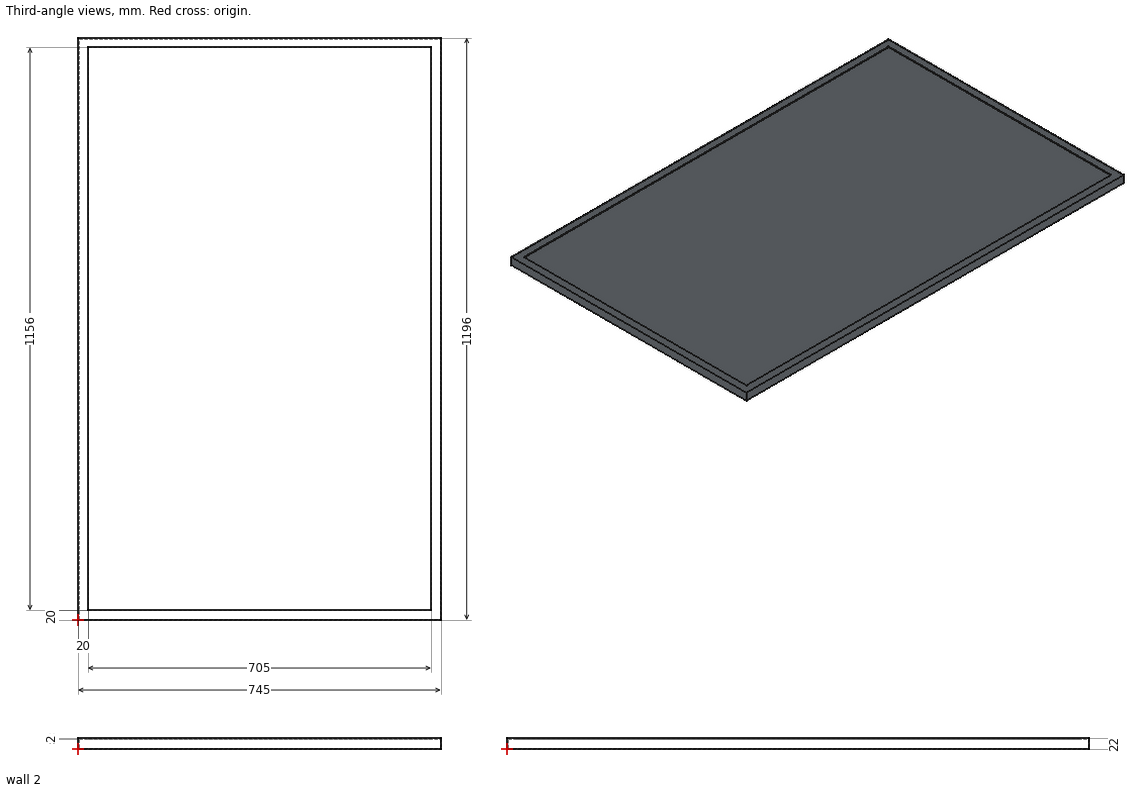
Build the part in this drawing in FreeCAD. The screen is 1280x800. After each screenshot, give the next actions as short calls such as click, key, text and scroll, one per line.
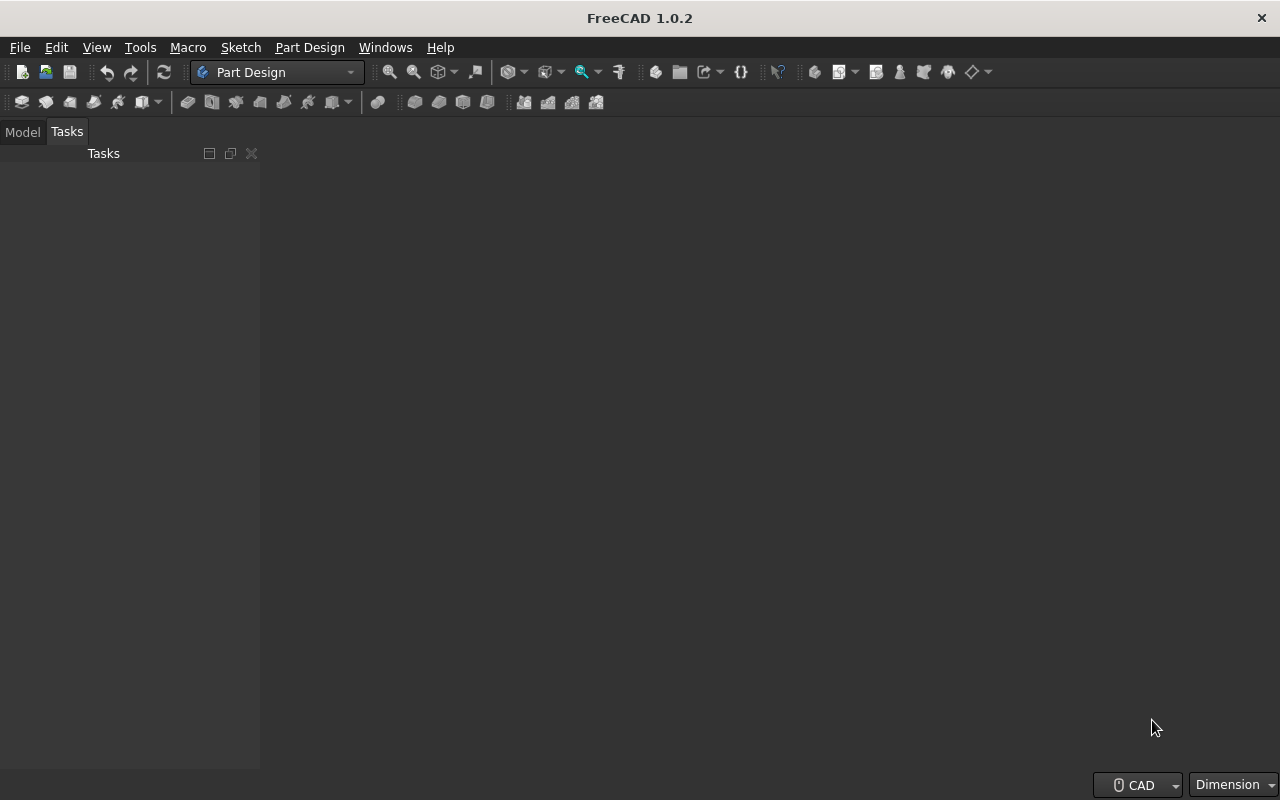
click(22, 72)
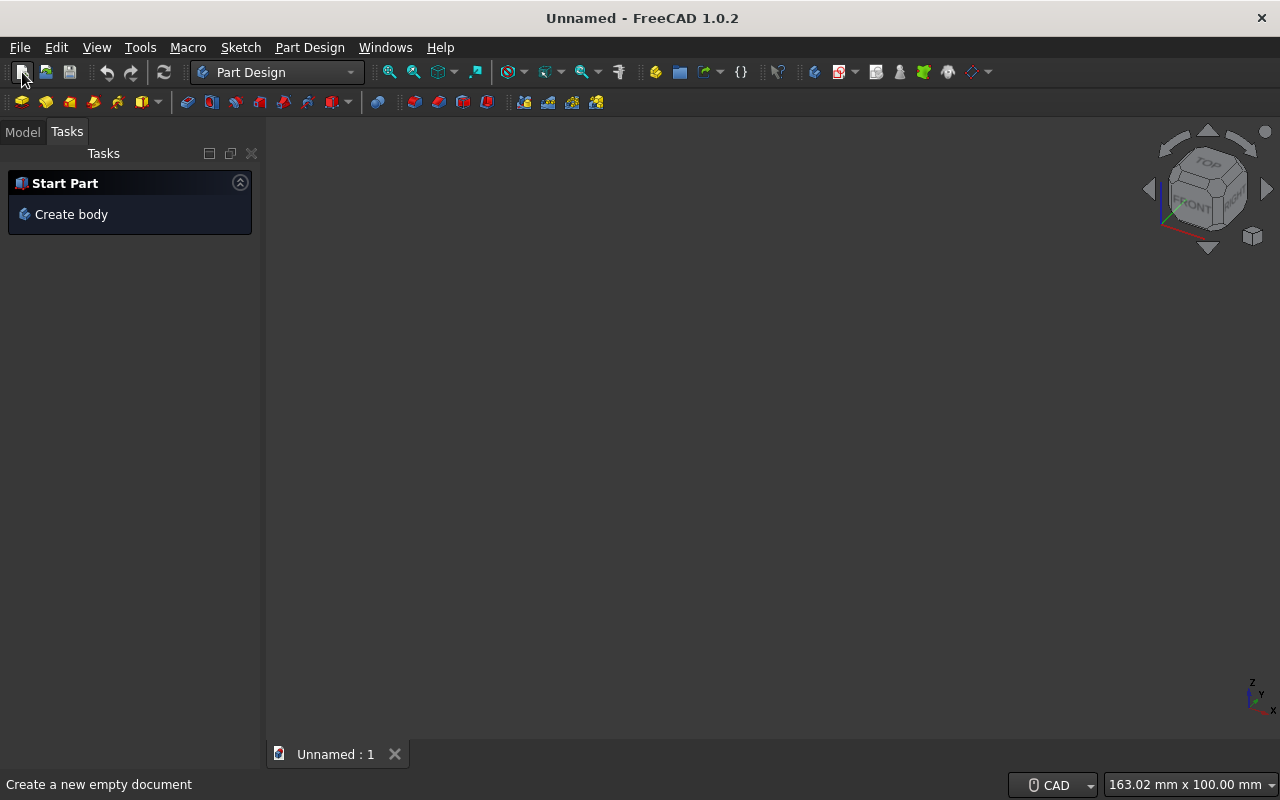
click(840, 72)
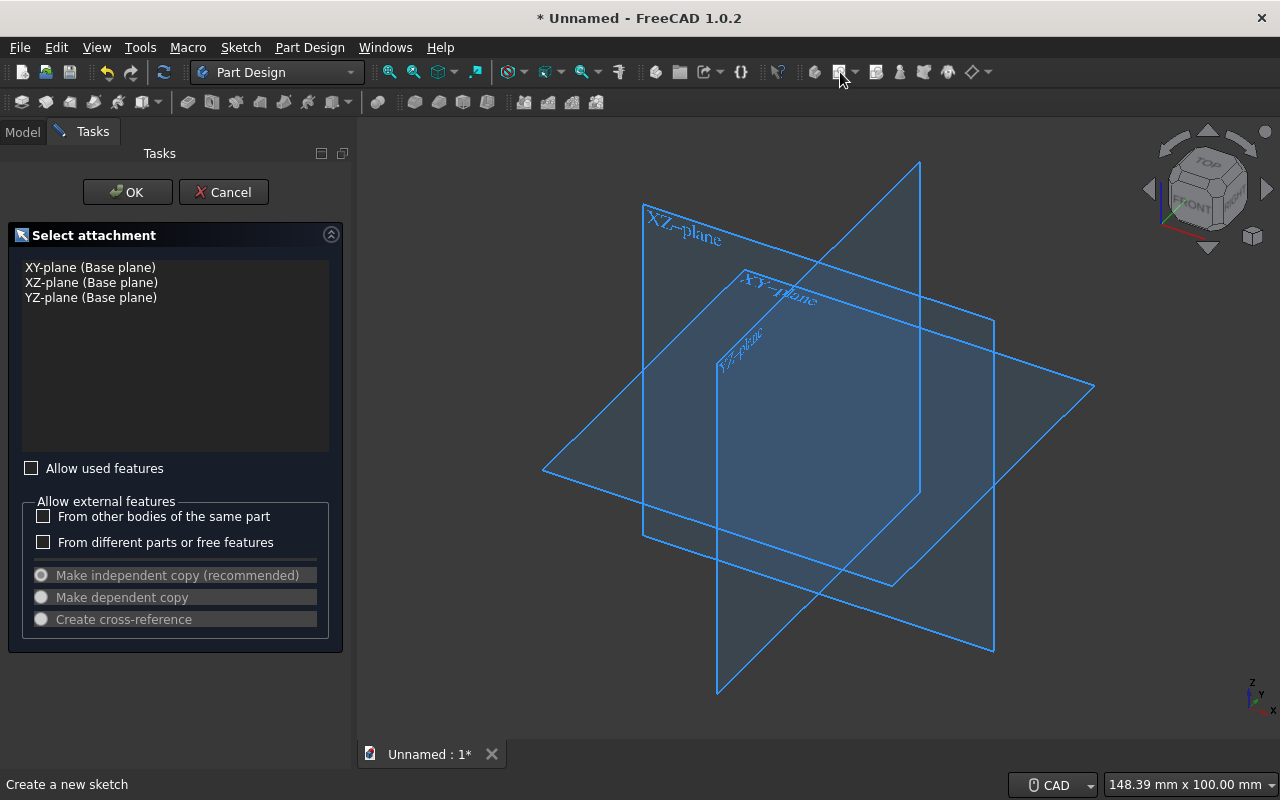
click(82, 268)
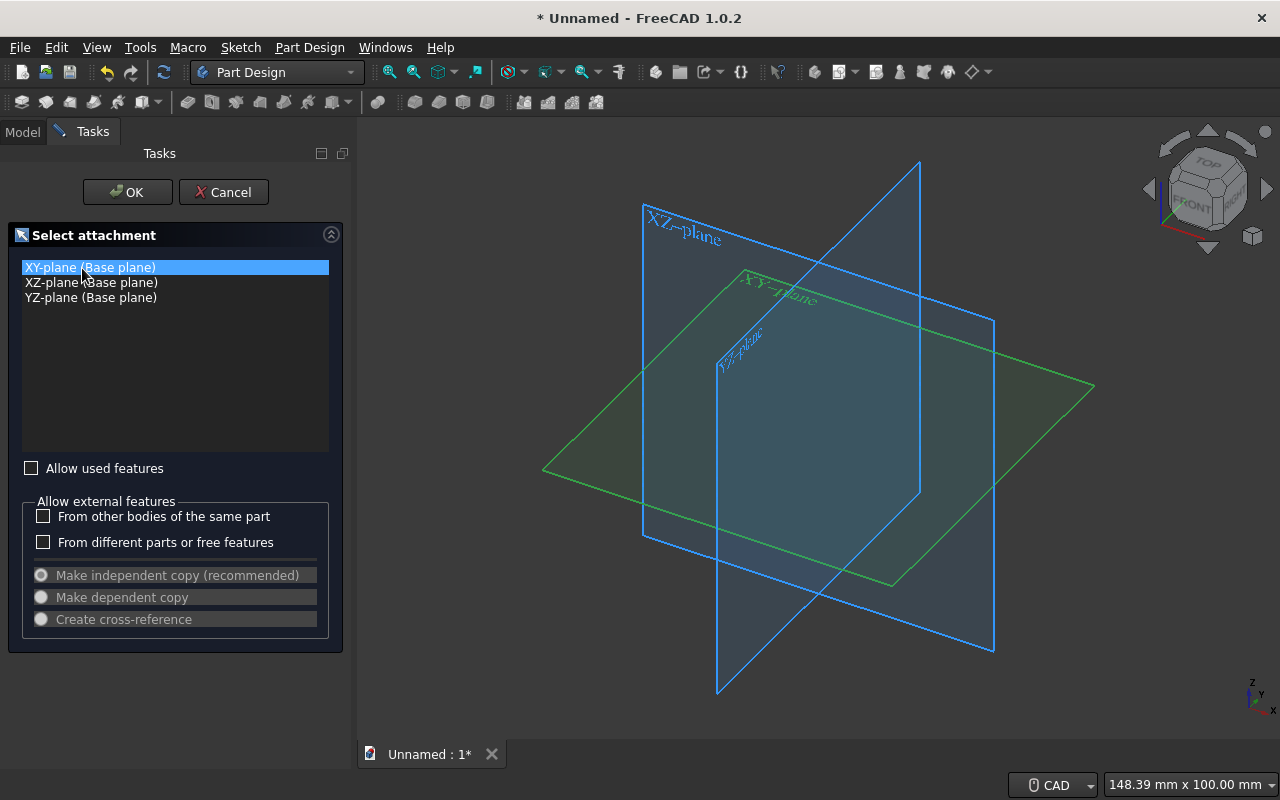
click(128, 192)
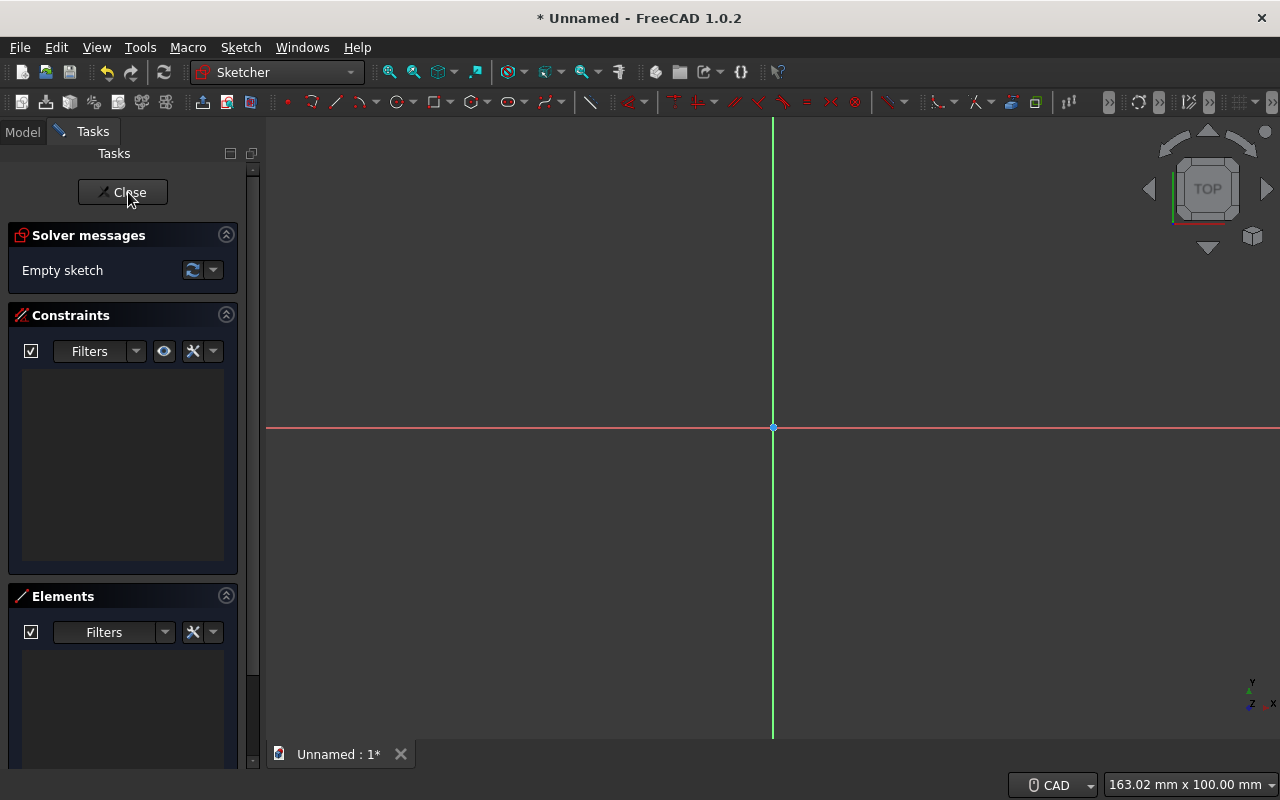
scroll(580, 623, down, 15)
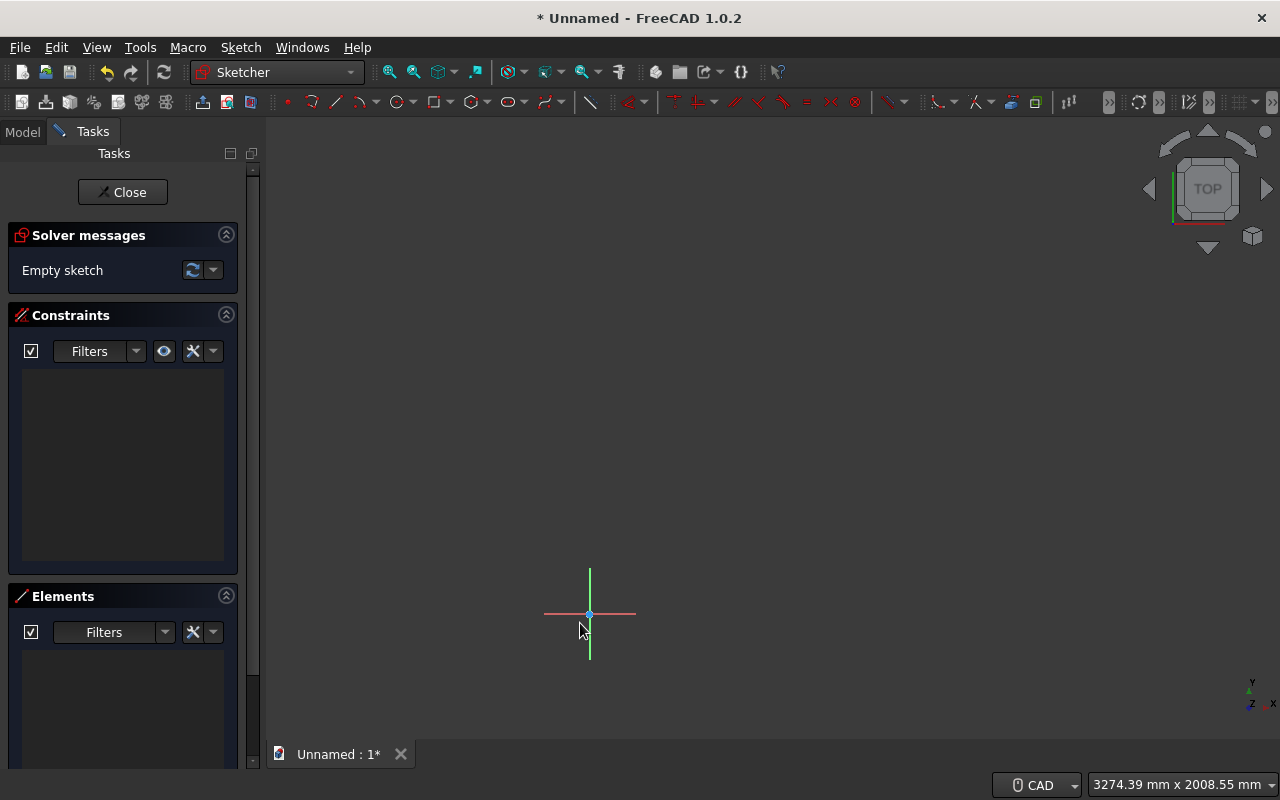
click(434, 102)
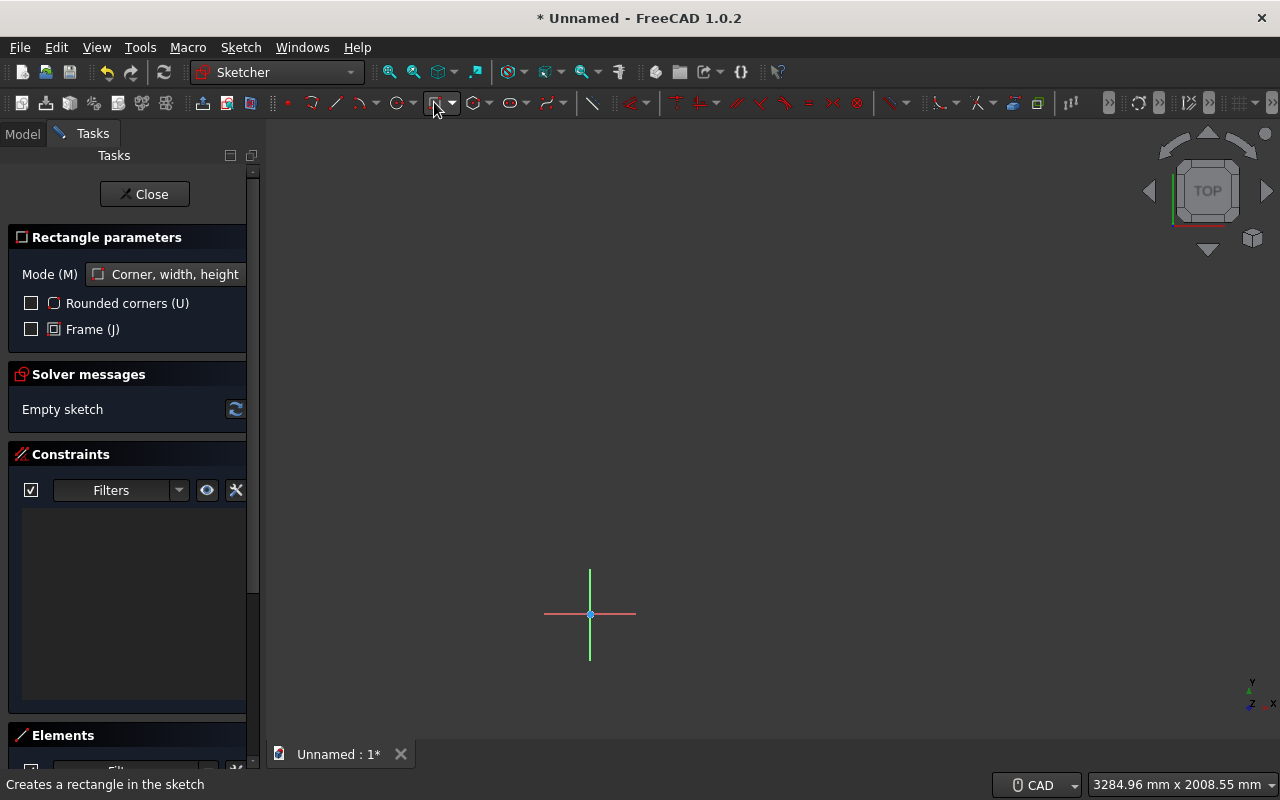
click(590, 614)
move(820, 245)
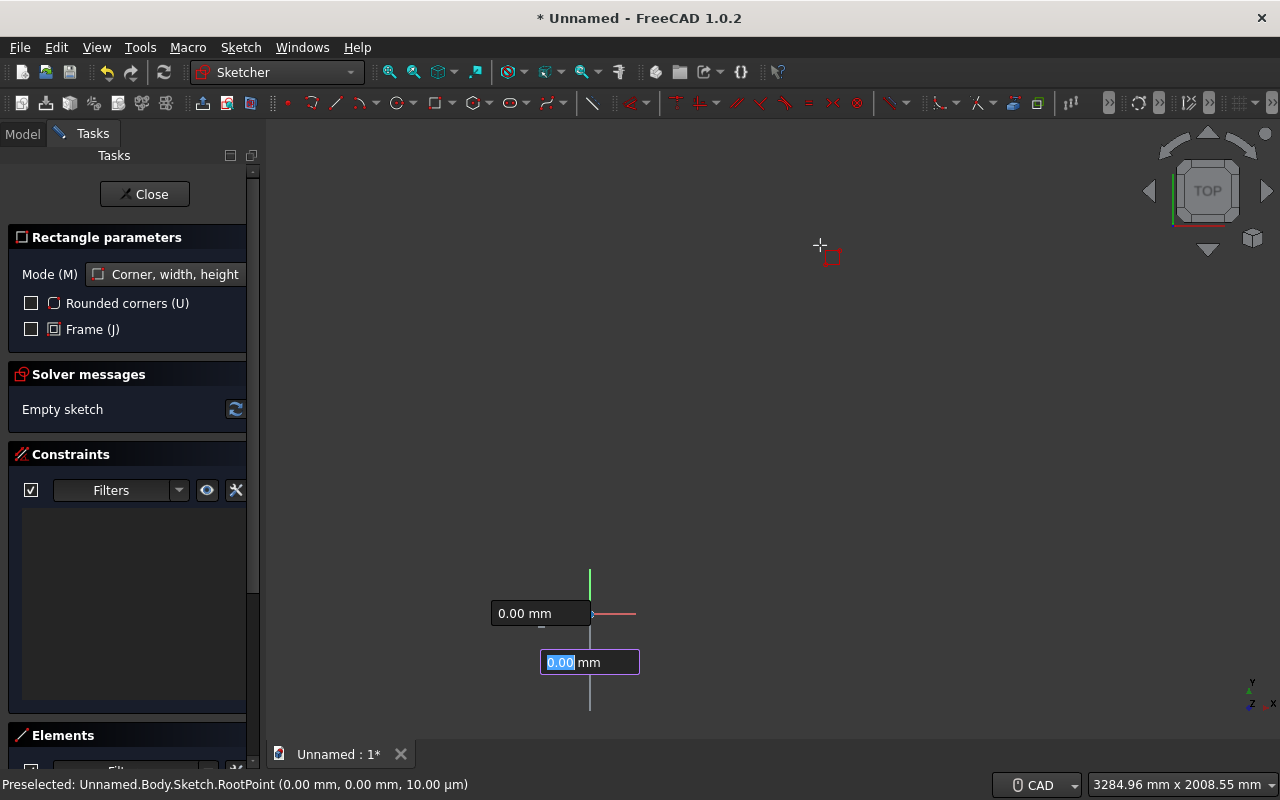
text(745)
key(Tab)
text(1196)
key(Return)
key(Escape)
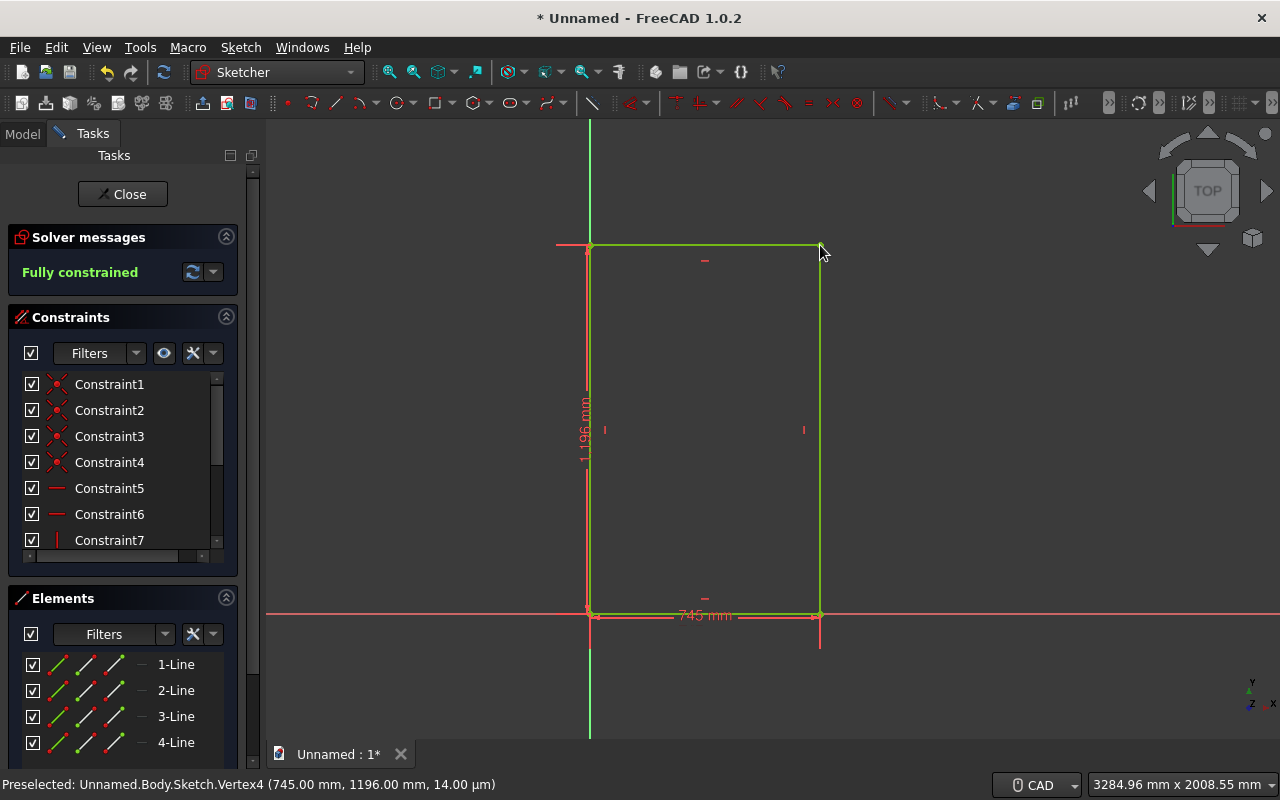
click(123, 194)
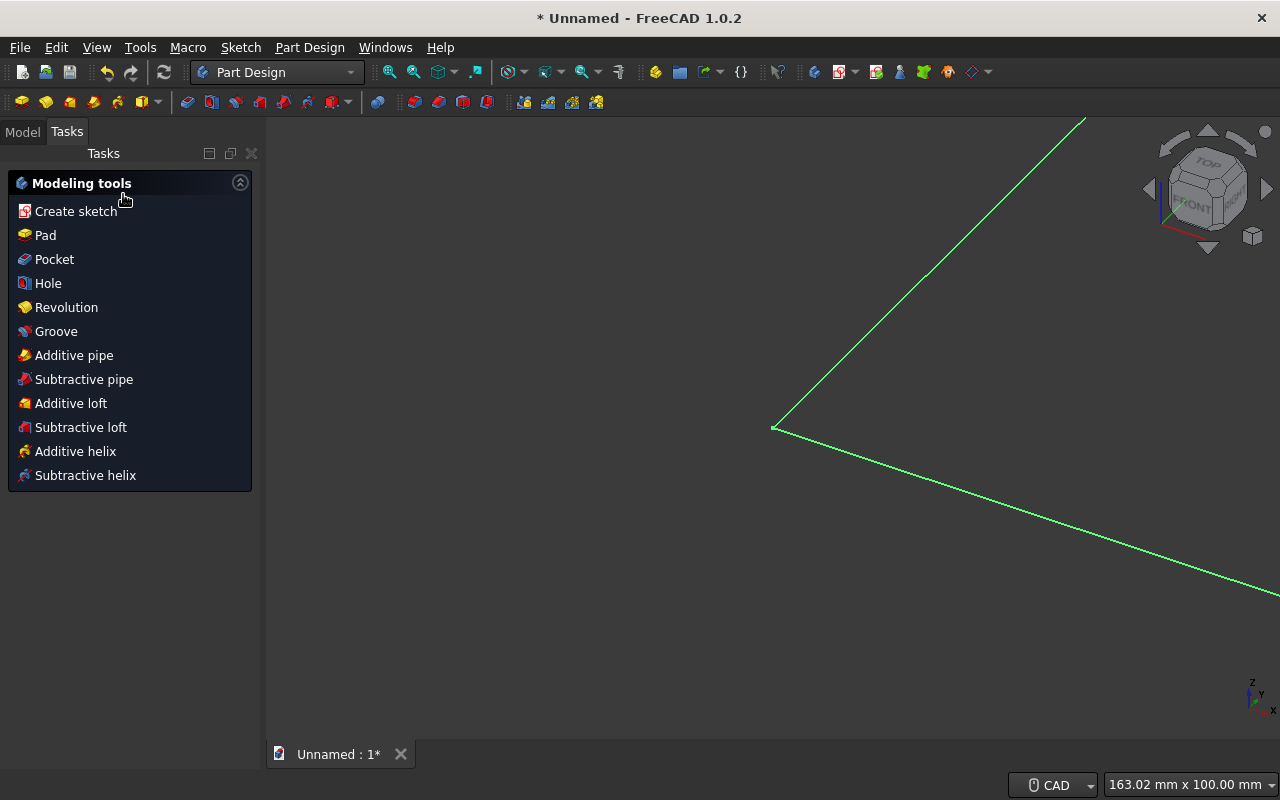
click(22, 102)